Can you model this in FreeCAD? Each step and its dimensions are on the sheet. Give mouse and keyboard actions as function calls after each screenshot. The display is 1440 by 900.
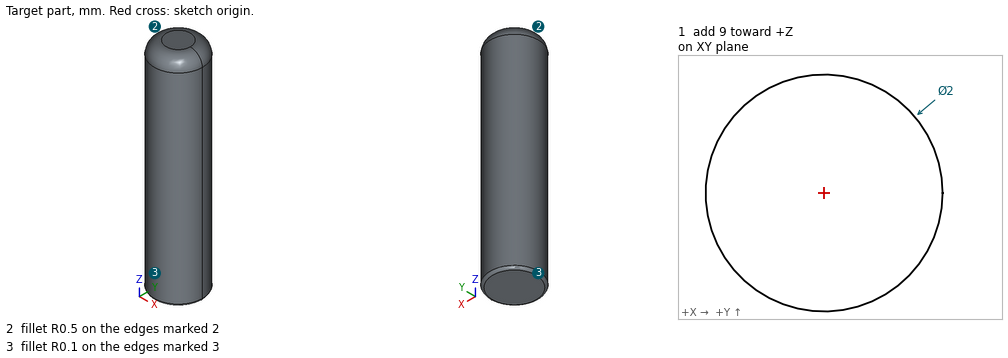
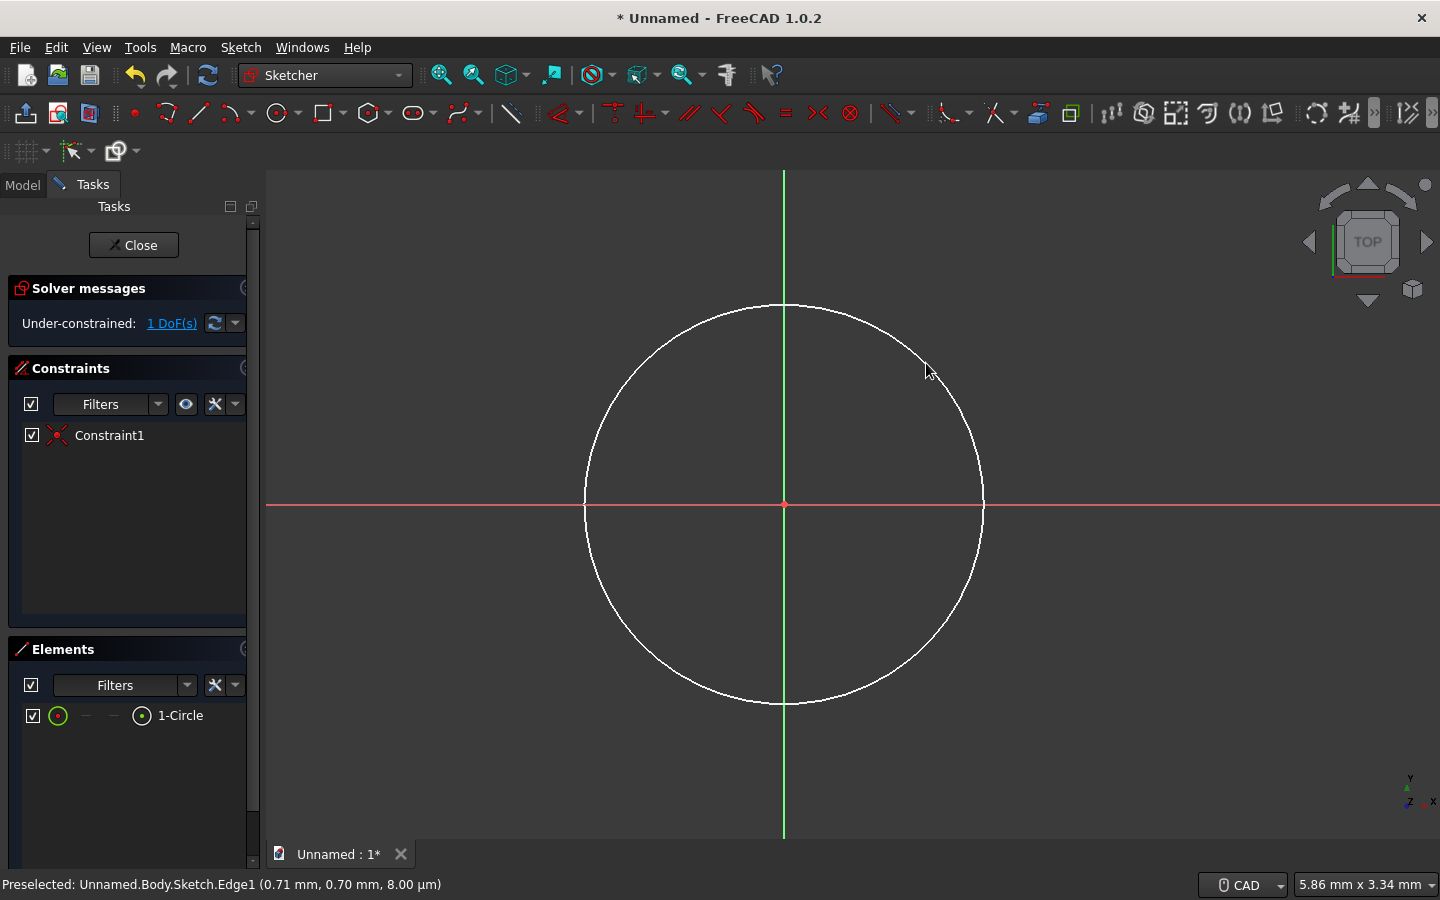
click(925, 363)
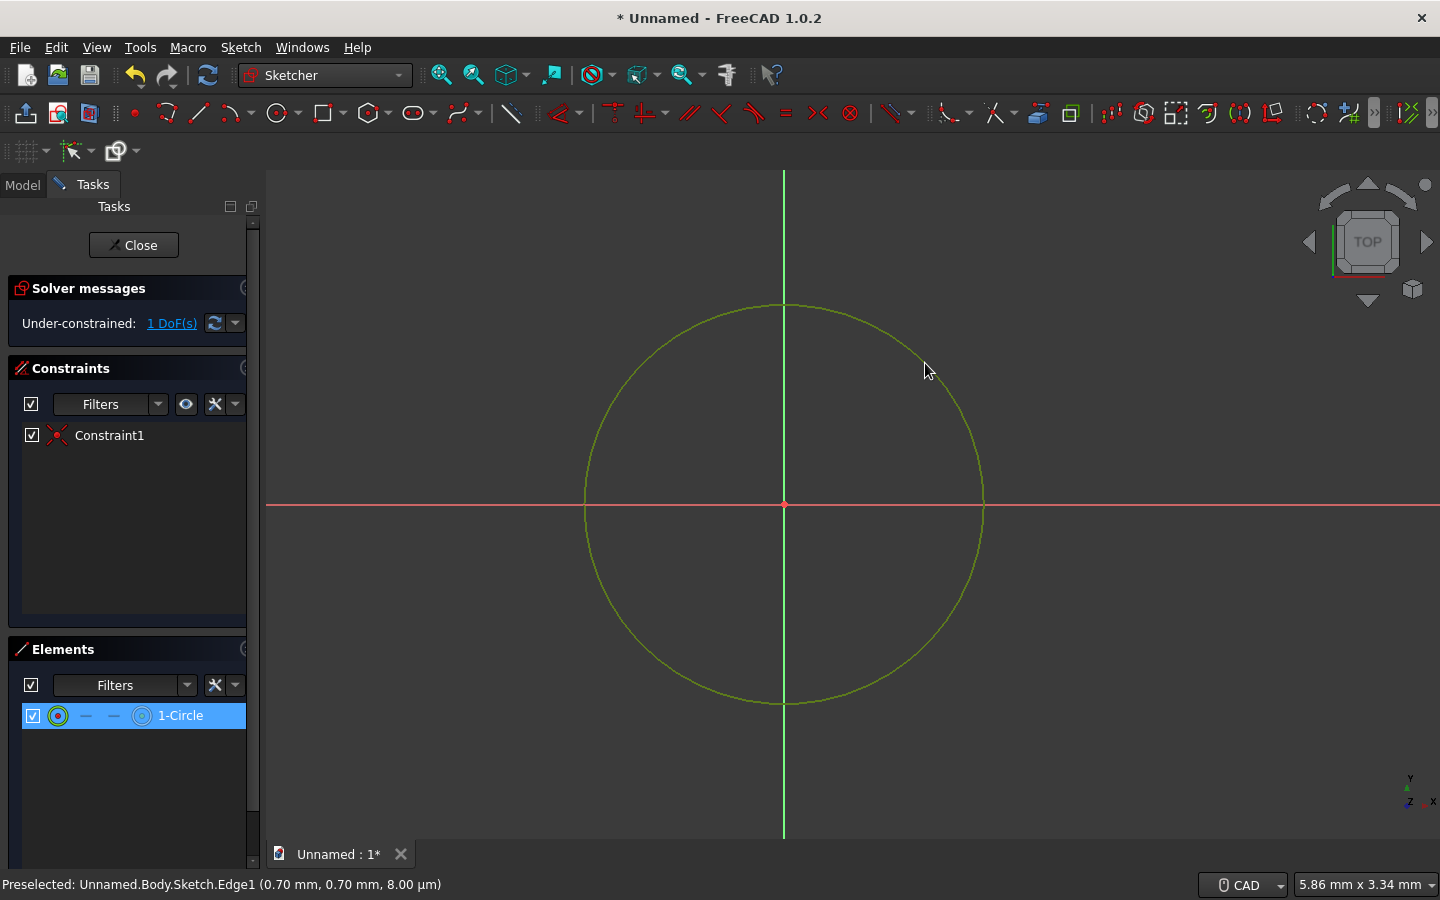
key(k)
key(o)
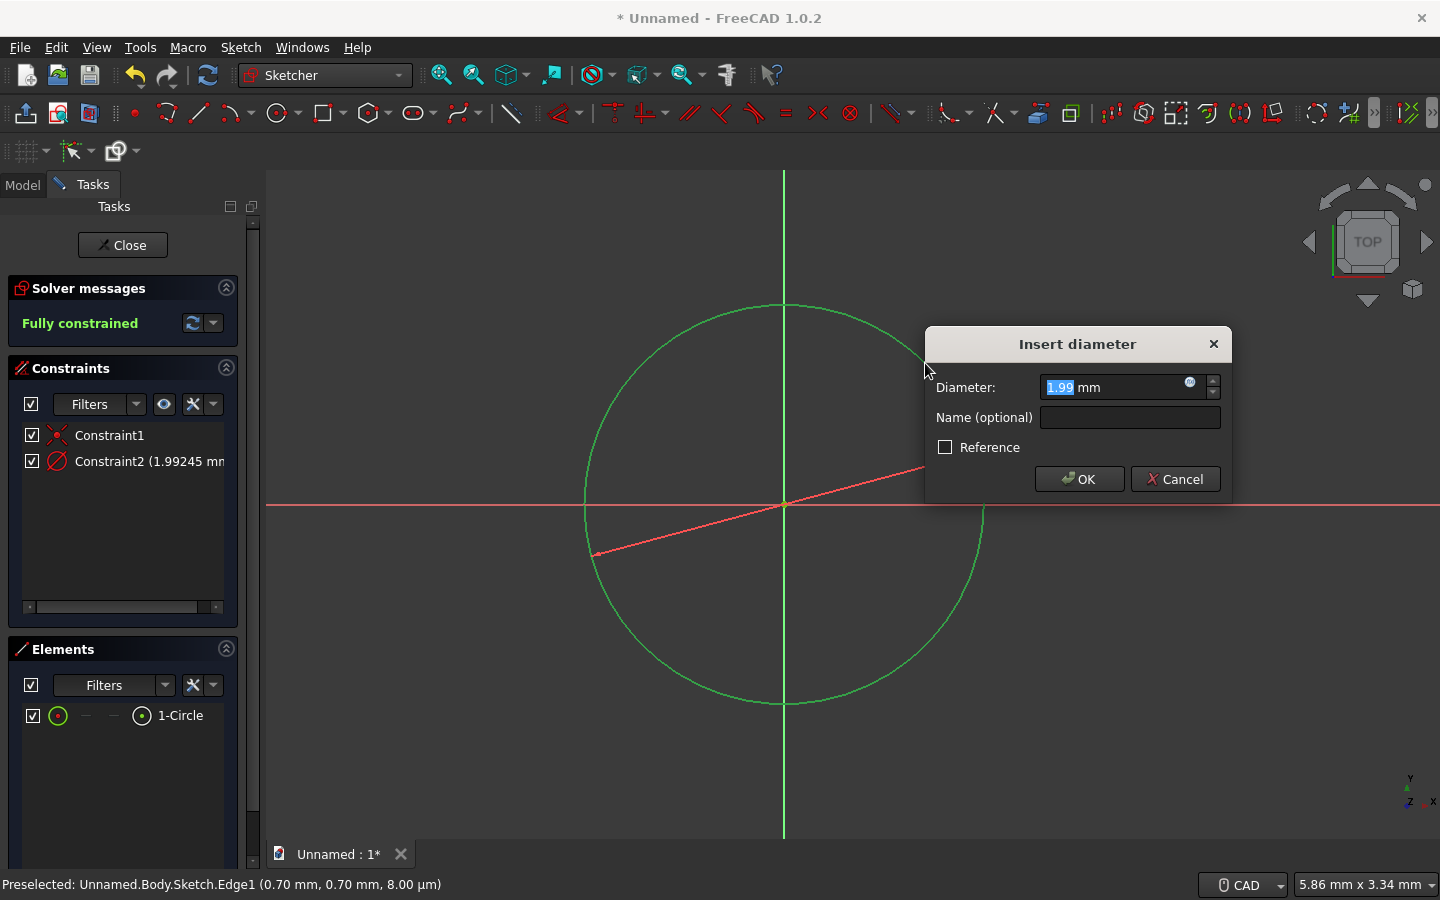
text(2)
key(Return)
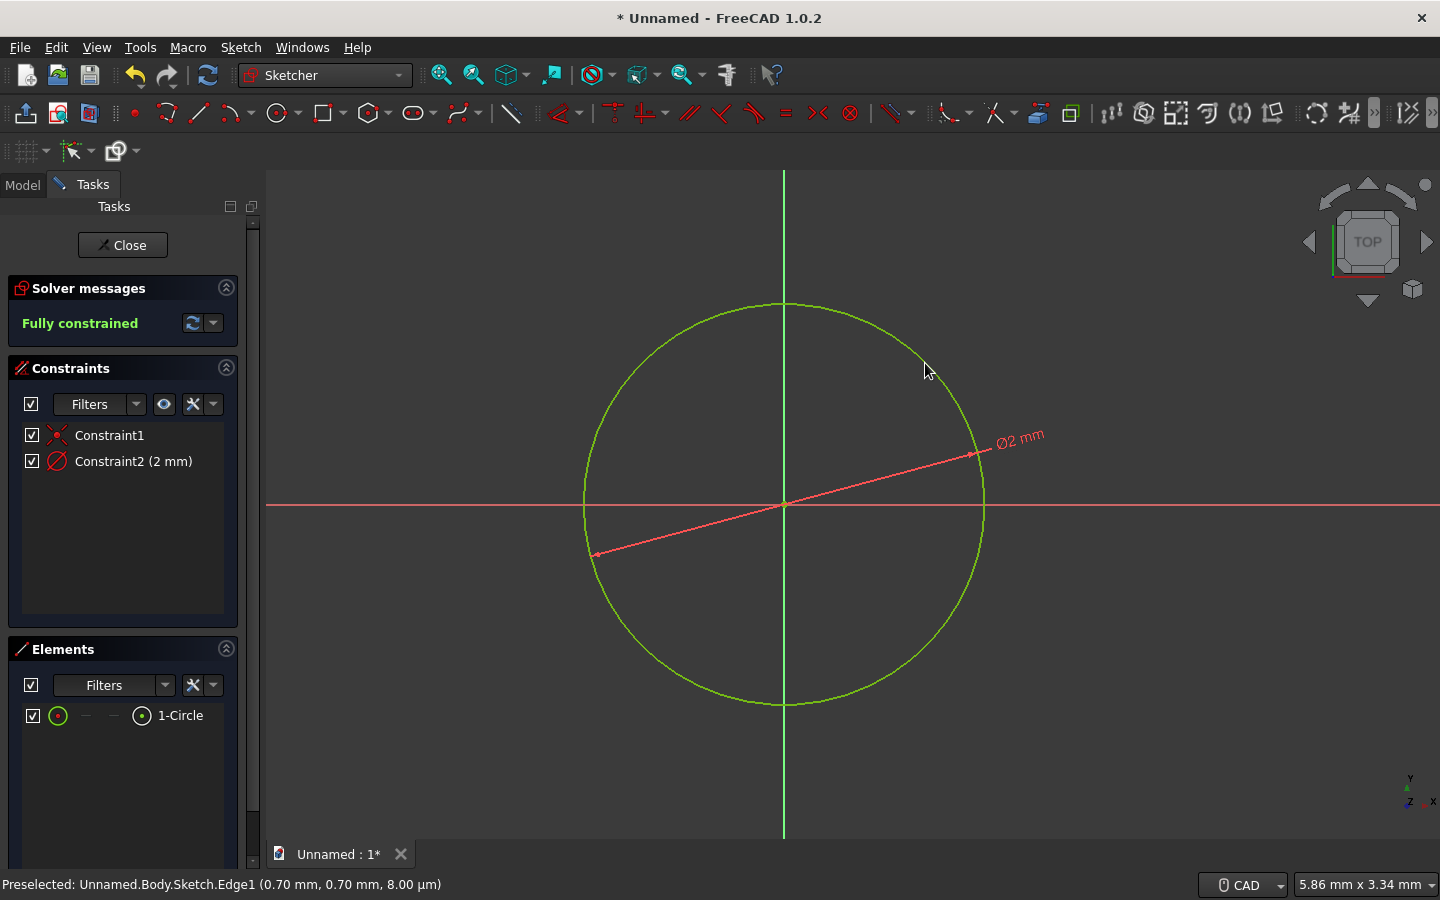
click(123, 245)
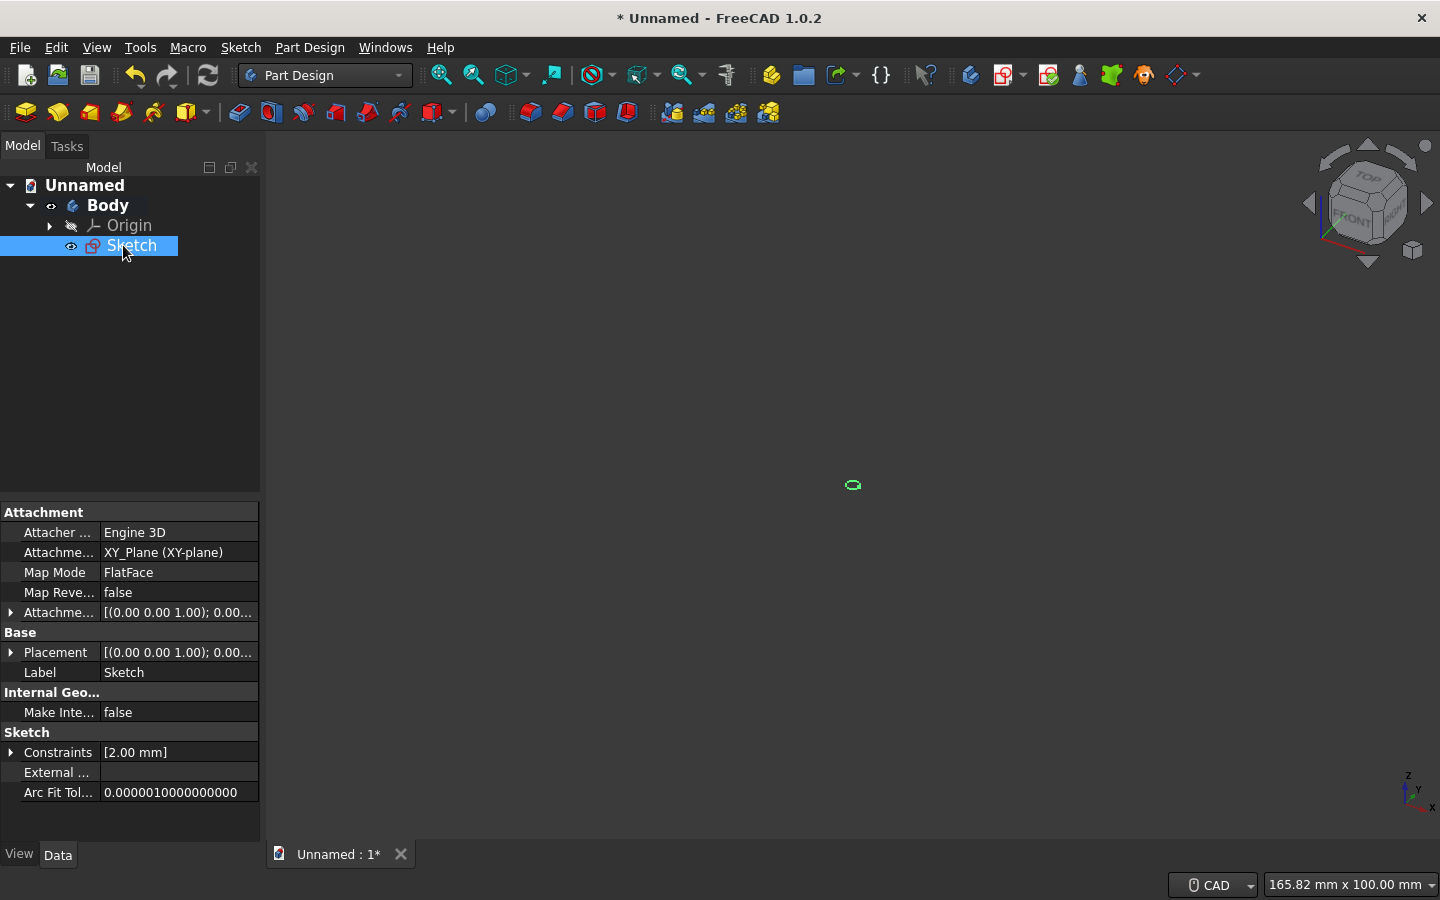
click(26, 112)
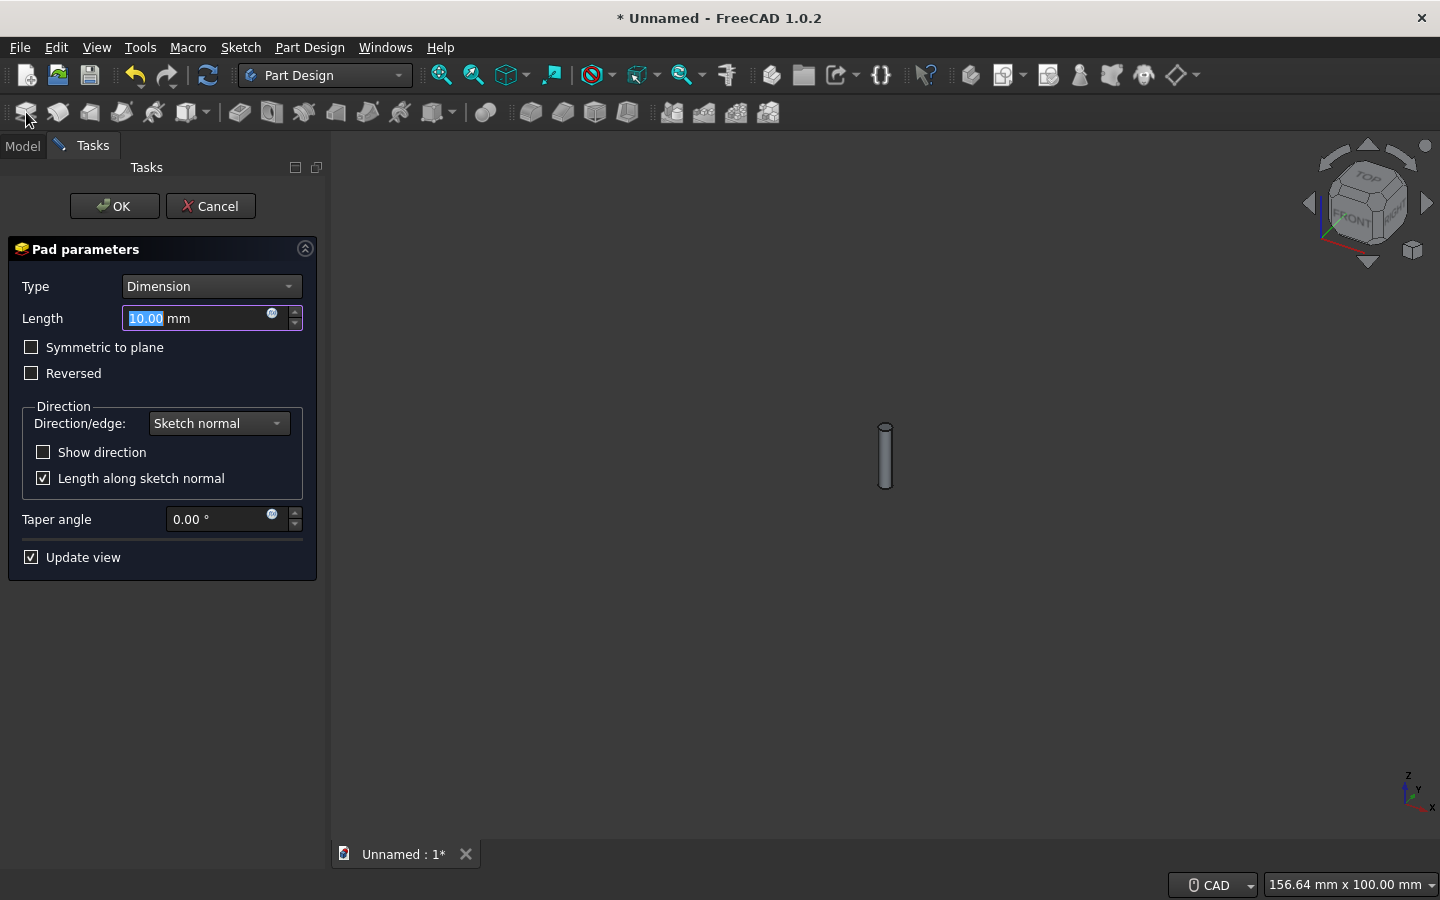
text(9)
key(Tab)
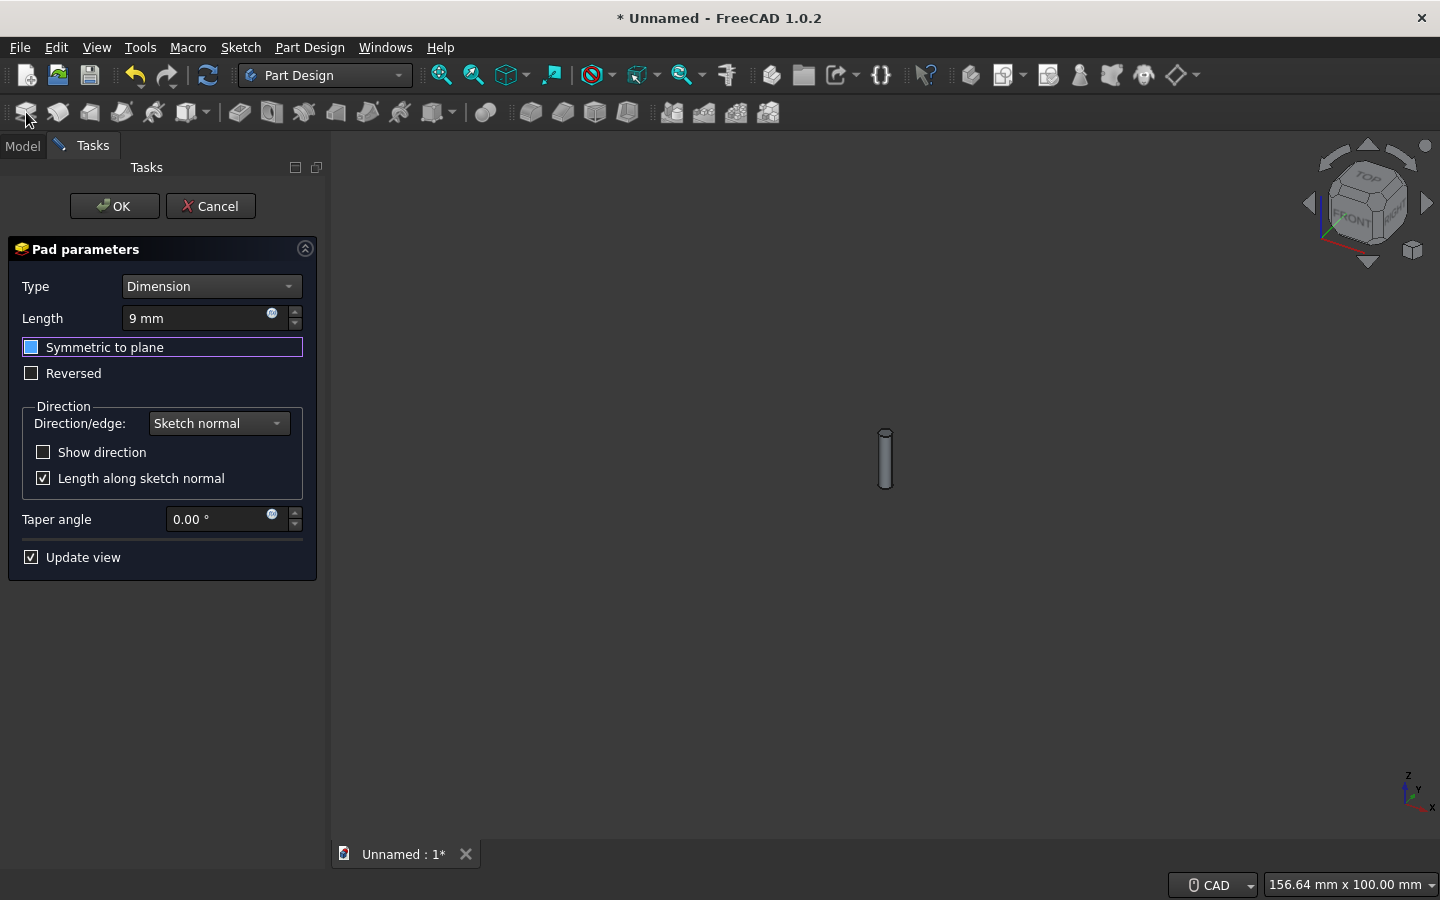
click(115, 206)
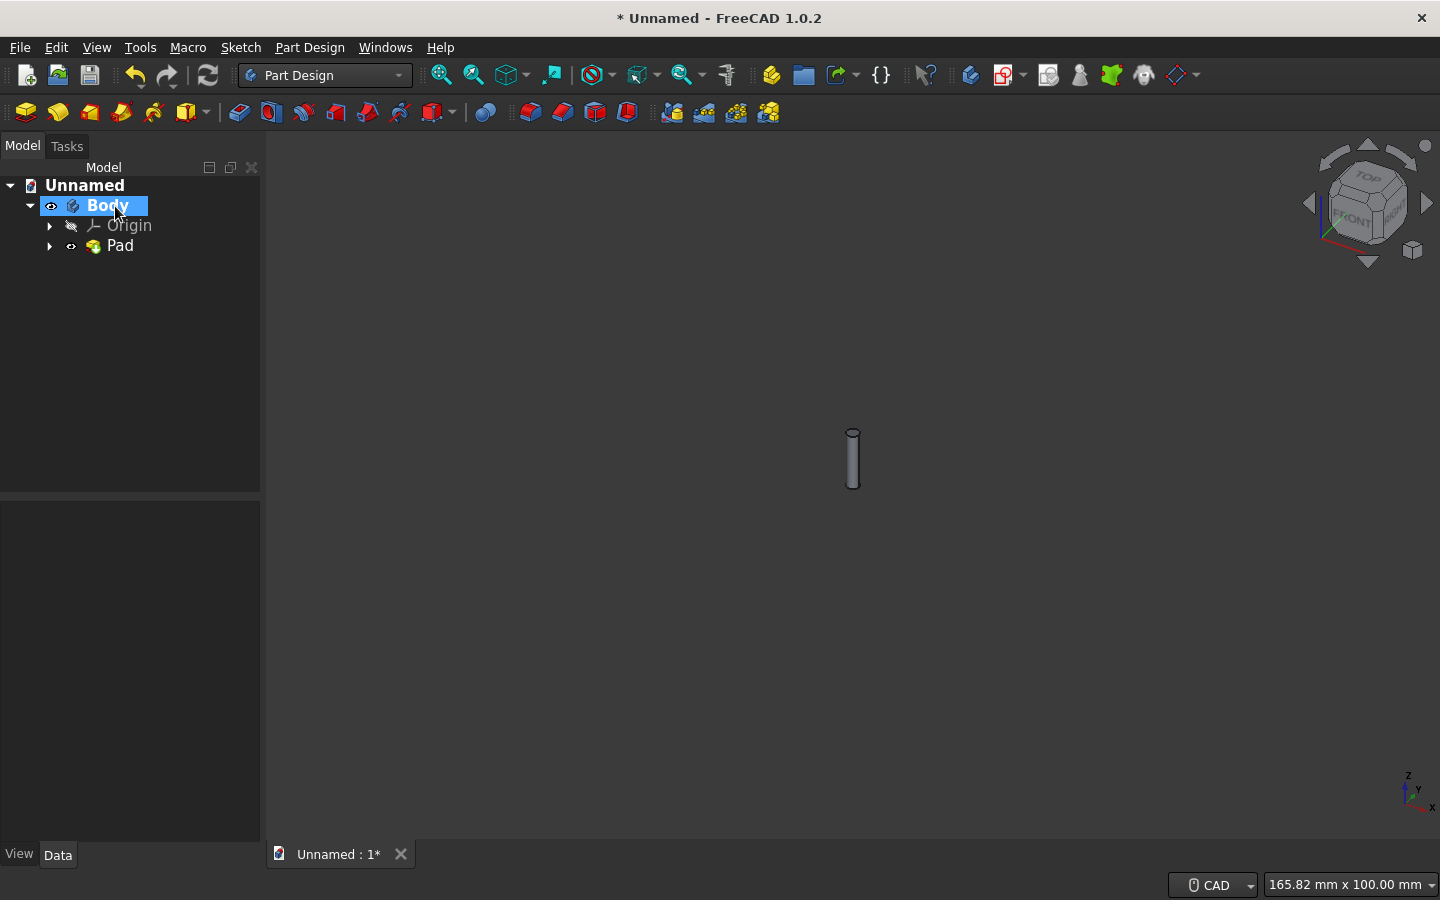
key(v)
key(f)